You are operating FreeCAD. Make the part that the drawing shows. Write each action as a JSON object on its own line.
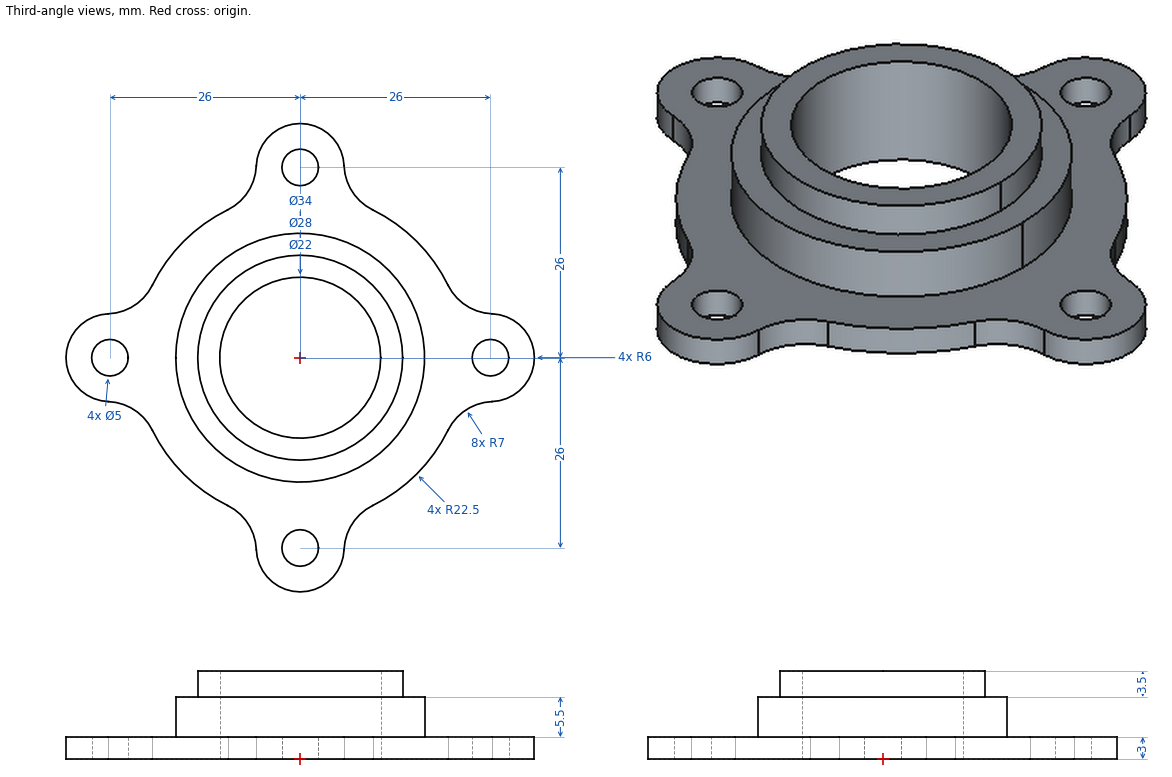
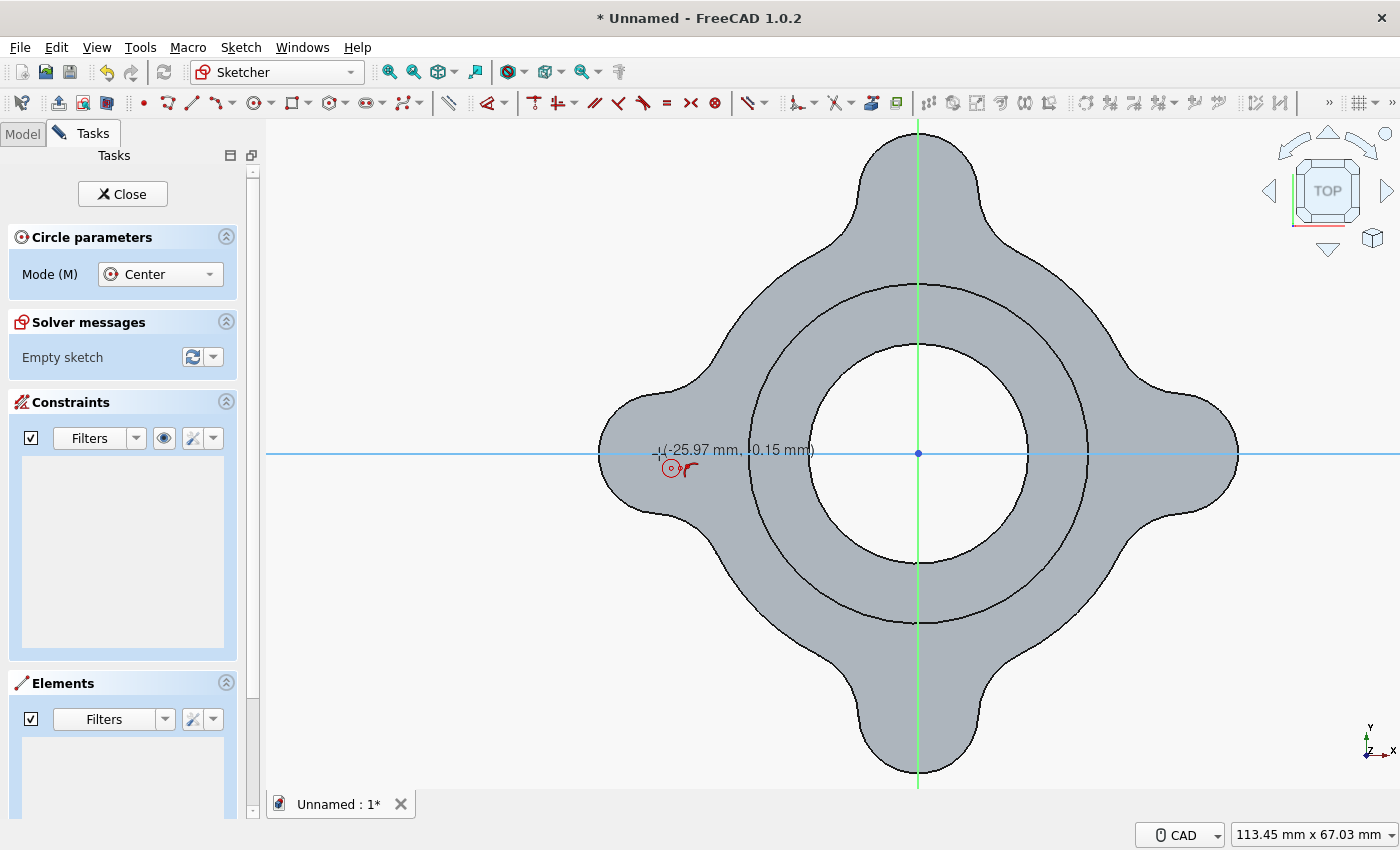
{"action": "left_click", "coordinate": [659, 454]}
{"action": "mouse_move", "coordinate": [676, 436]}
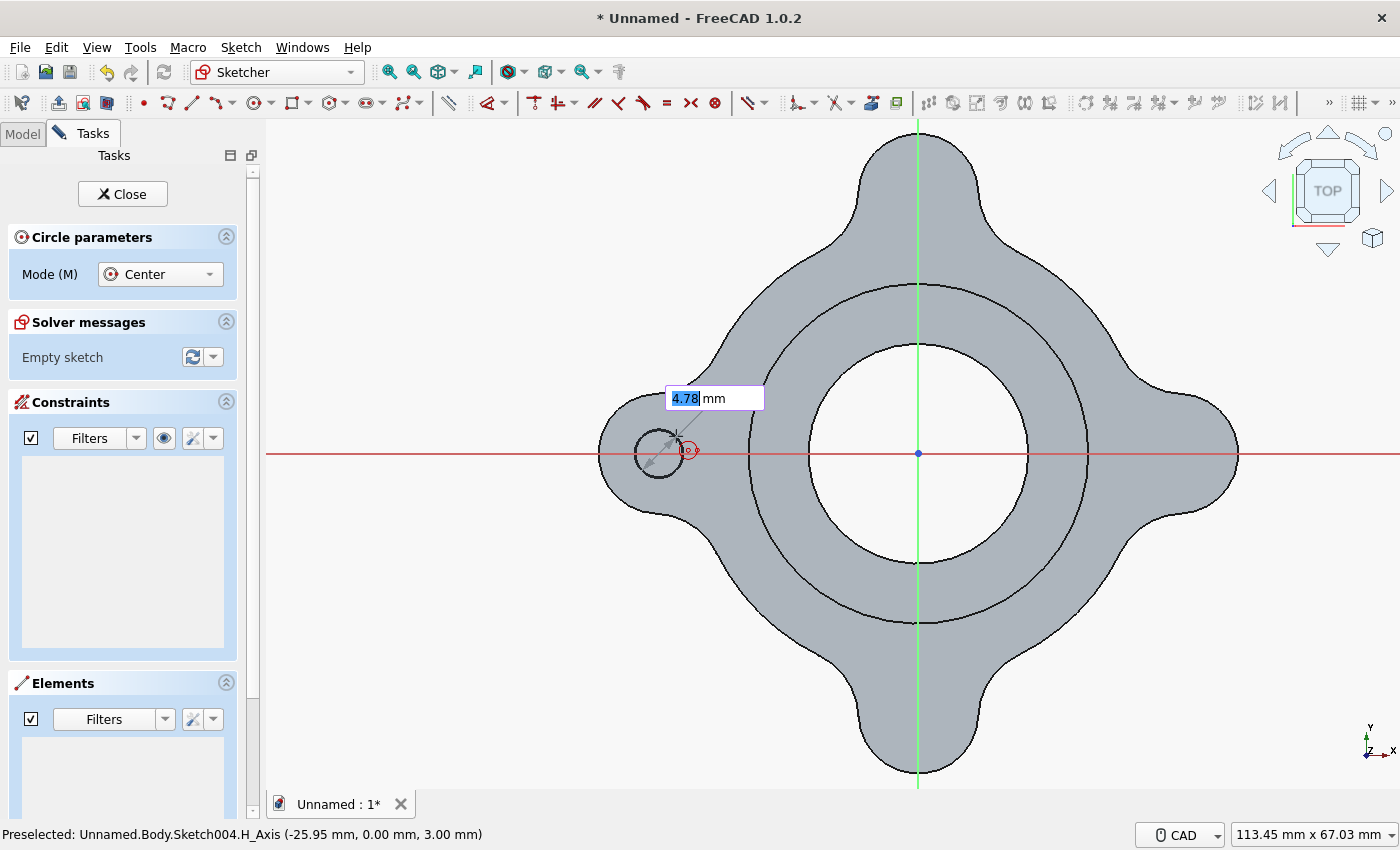
{"action": "type", "text": "5"}
{"action": "key", "text": "Return"}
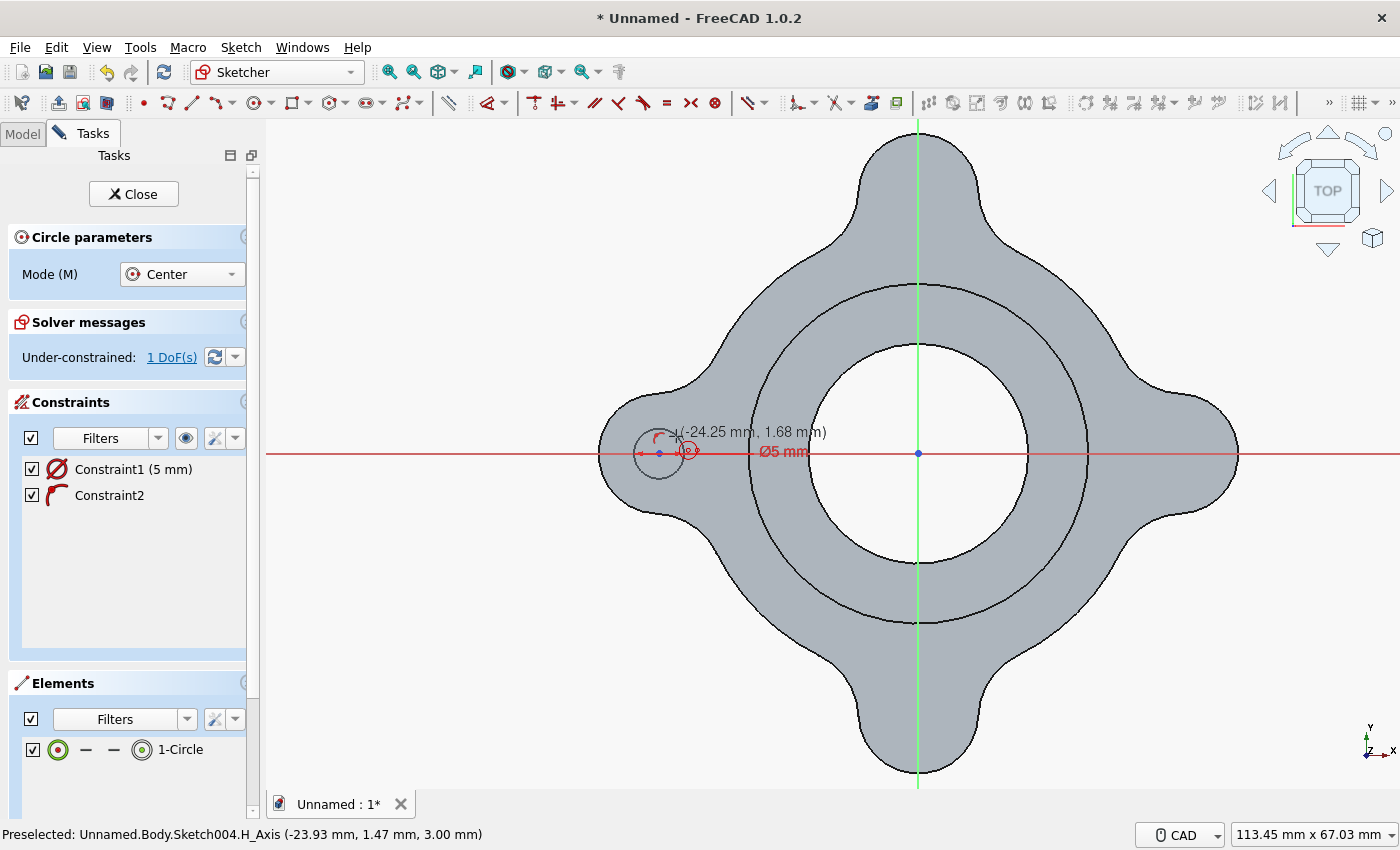
{"action": "left_click", "coordinate": [918, 194]}
{"action": "mouse_move", "coordinate": [936, 176]}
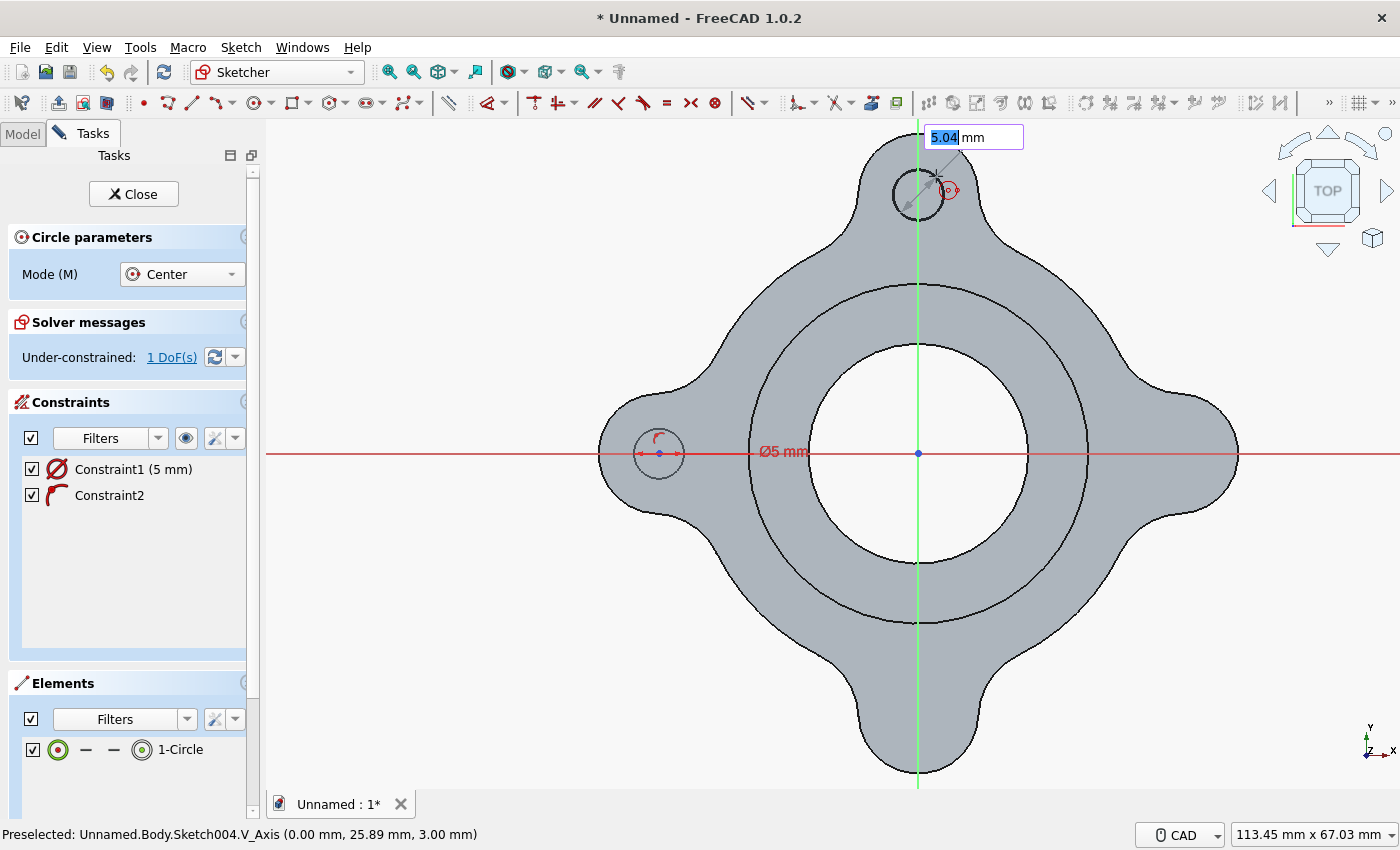
{"action": "type", "text": "5"}
{"action": "key", "text": "Return"}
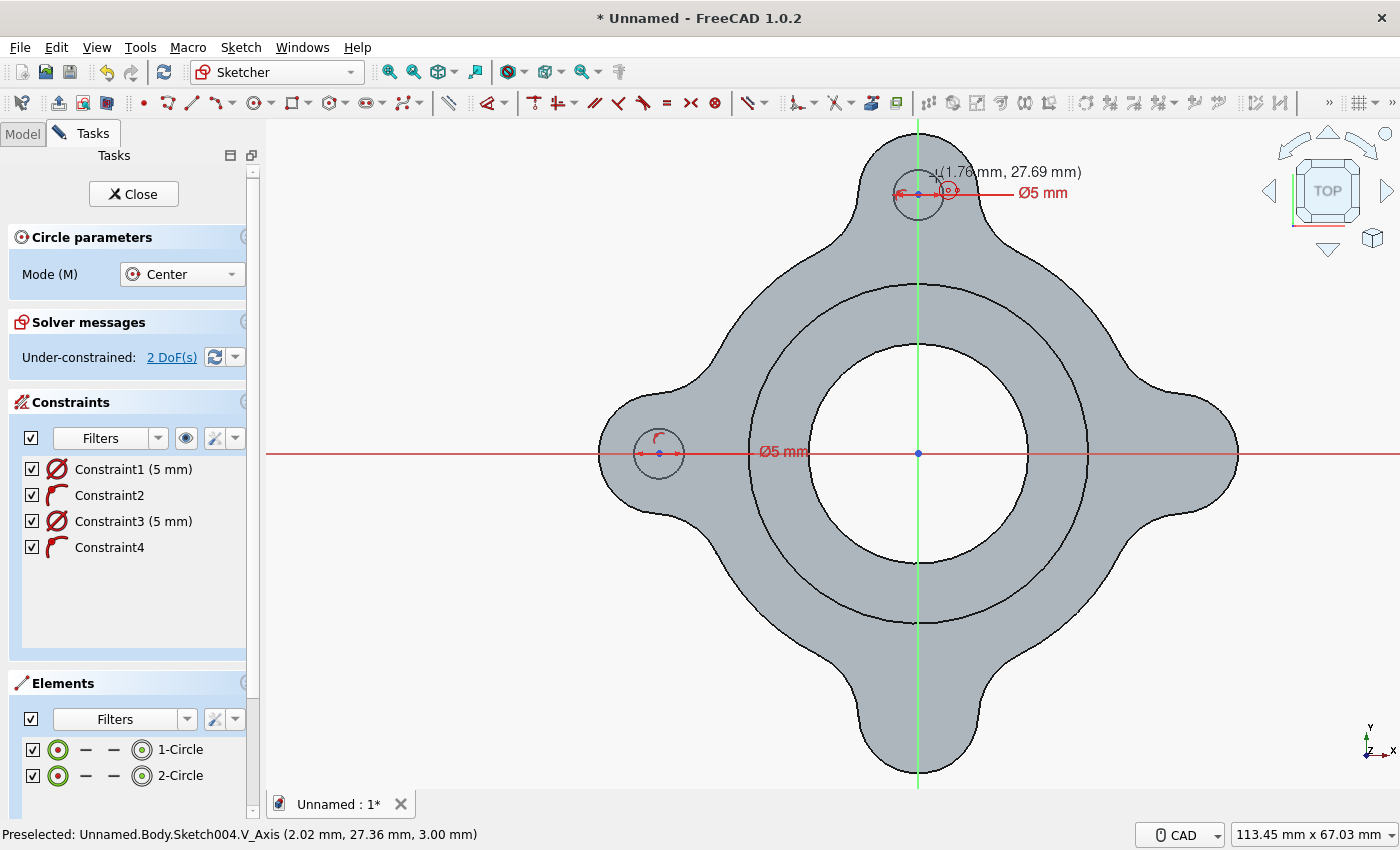
{"action": "left_click", "coordinate": [1178, 454]}
{"action": "mouse_move", "coordinate": [1196, 436]}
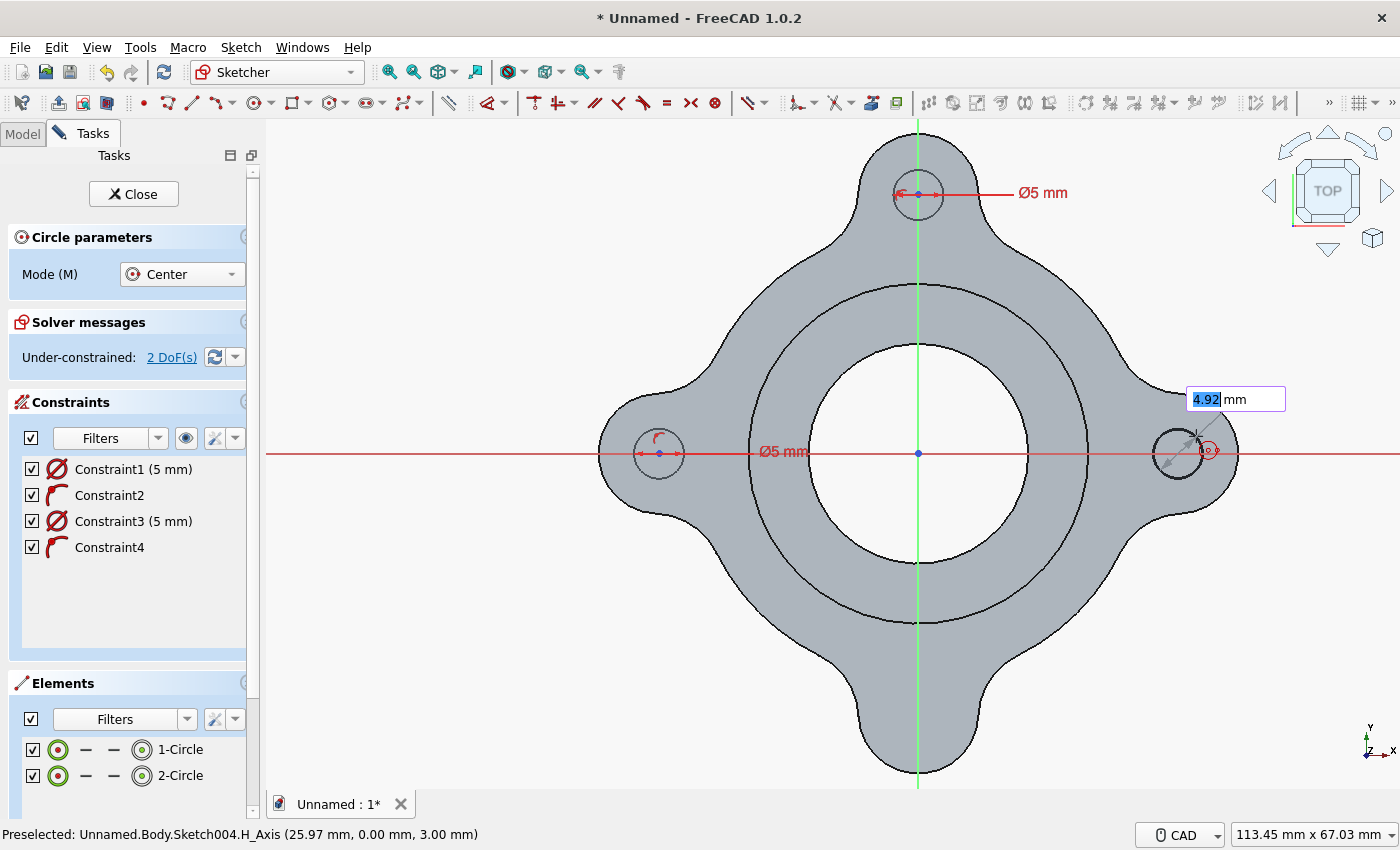
{"action": "type", "text": "5"}
{"action": "key", "text": "Return"}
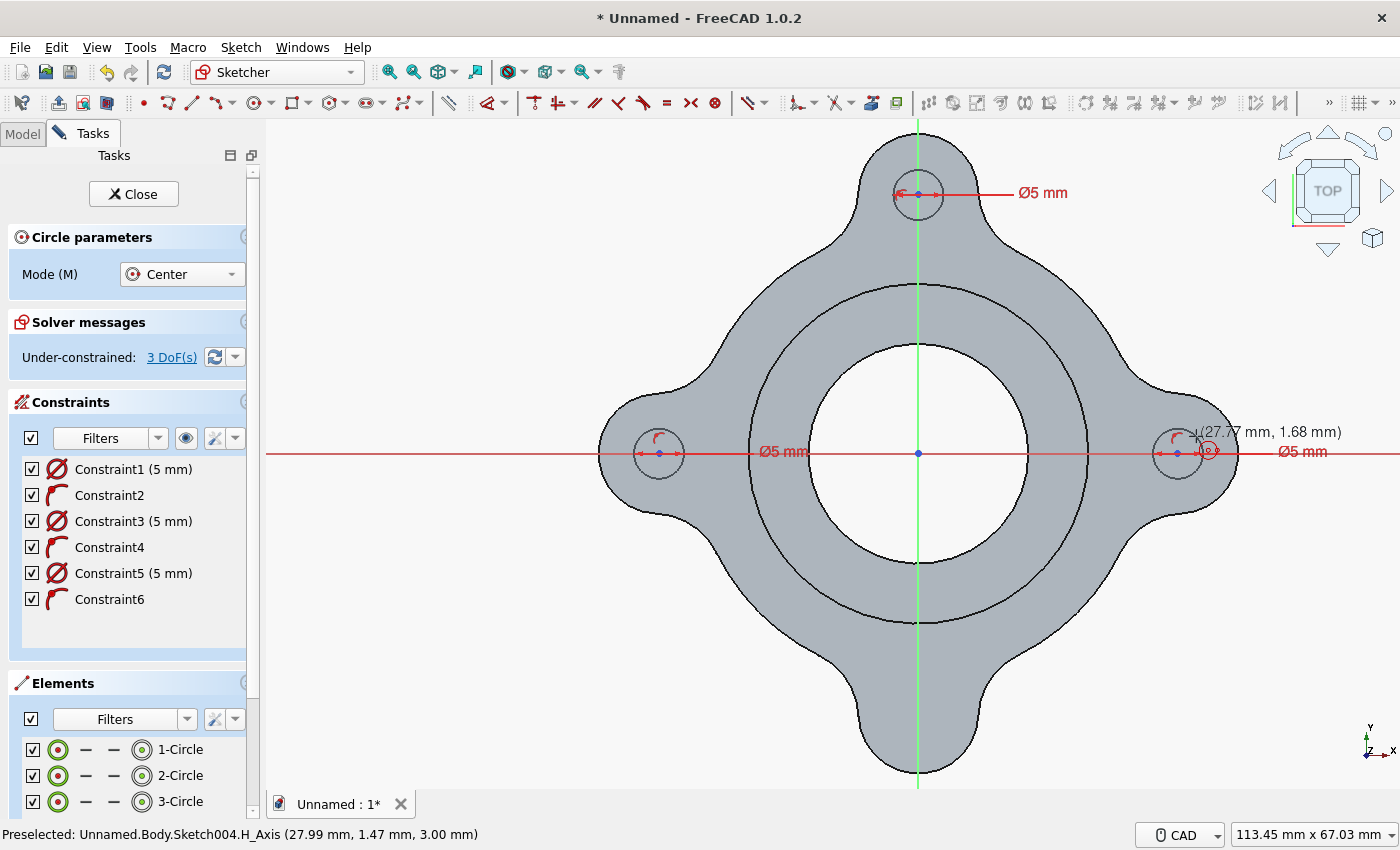
{"action": "left_click", "coordinate": [918, 714]}
{"action": "mouse_move", "coordinate": [936, 696]}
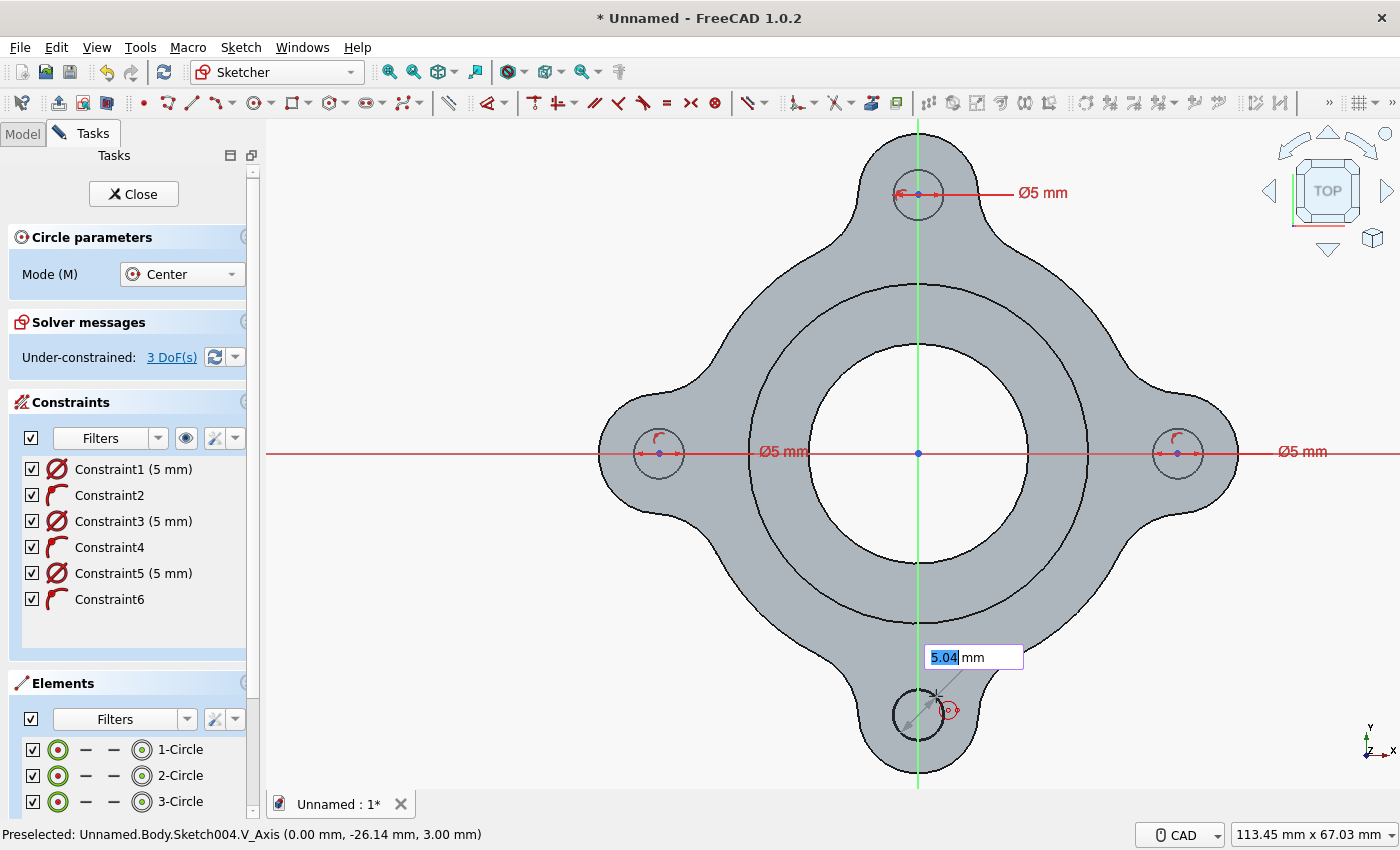
{"action": "type", "text": "5"}
{"action": "key", "text": "Return"}
{"action": "key", "text": "Escape"}